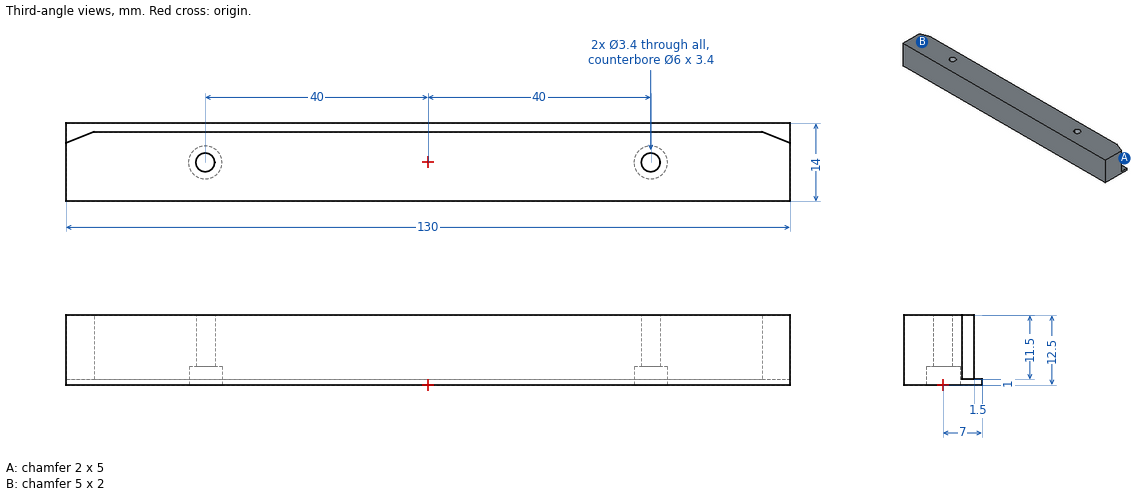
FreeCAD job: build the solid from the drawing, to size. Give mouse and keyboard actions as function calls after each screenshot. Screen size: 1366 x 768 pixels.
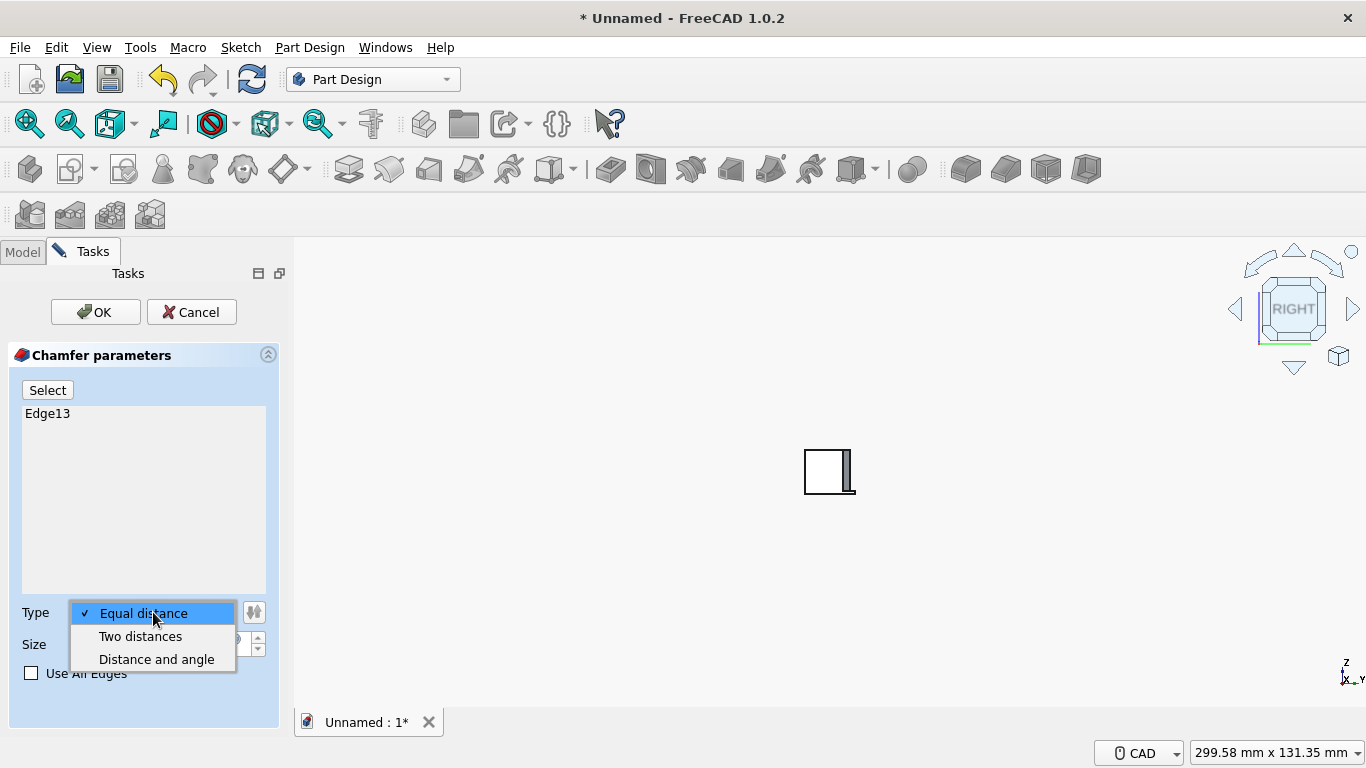
click(152, 636)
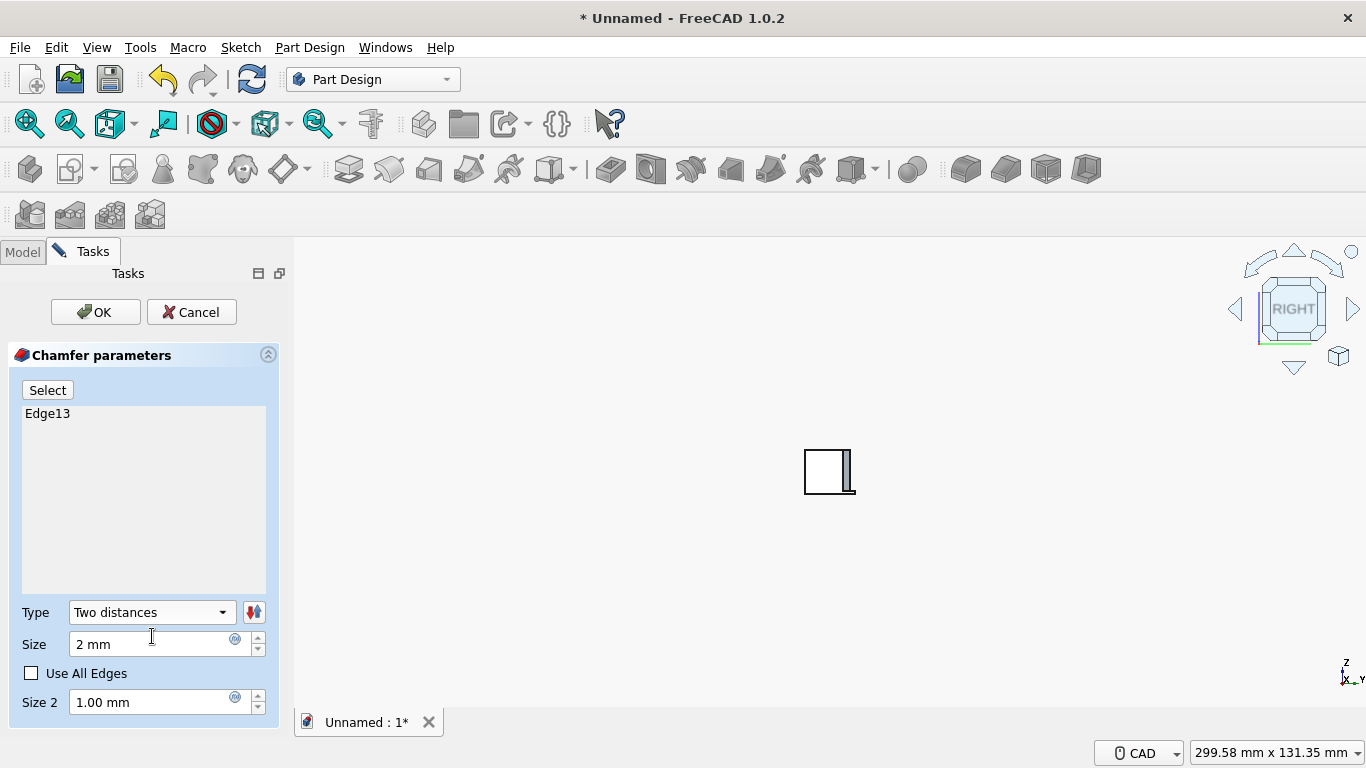
triple_click(160, 702)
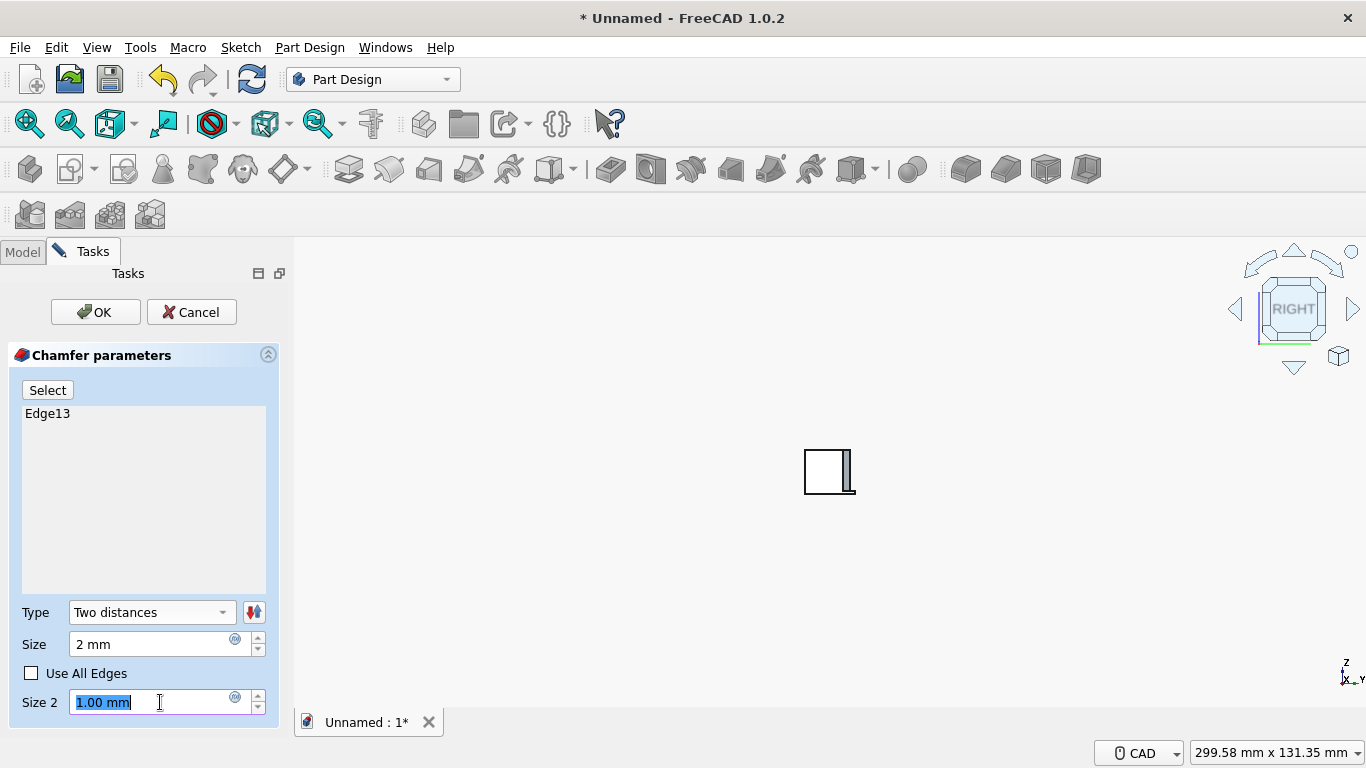
text(5)
key(Tab)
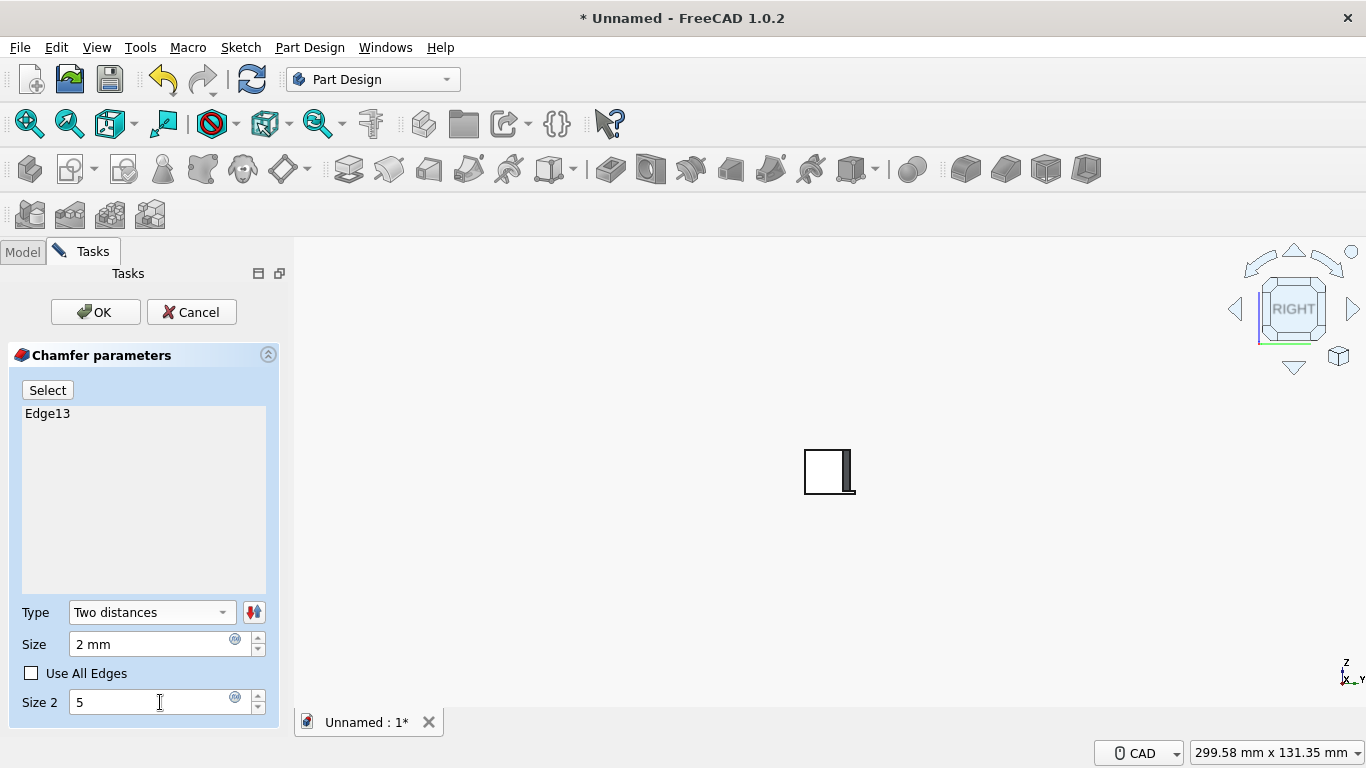
click(96, 312)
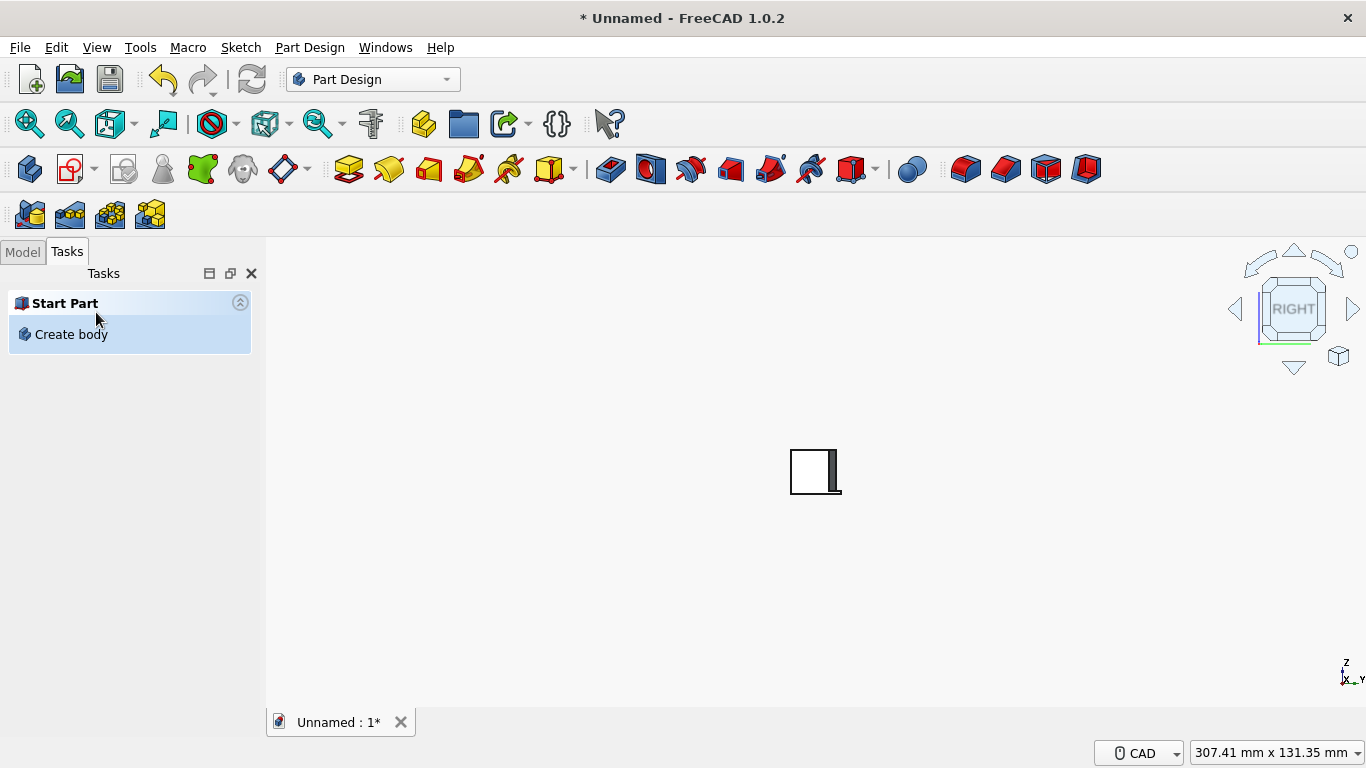
click(30, 124)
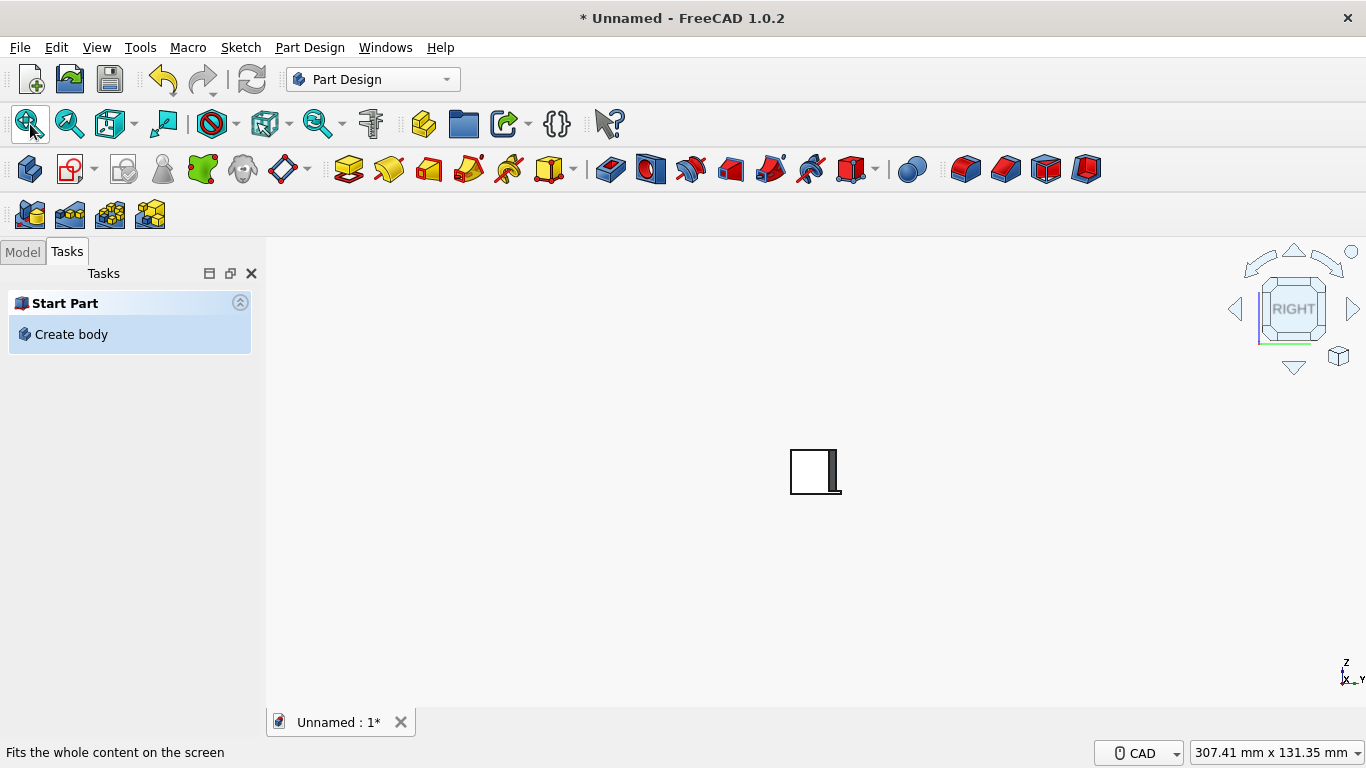
key(0)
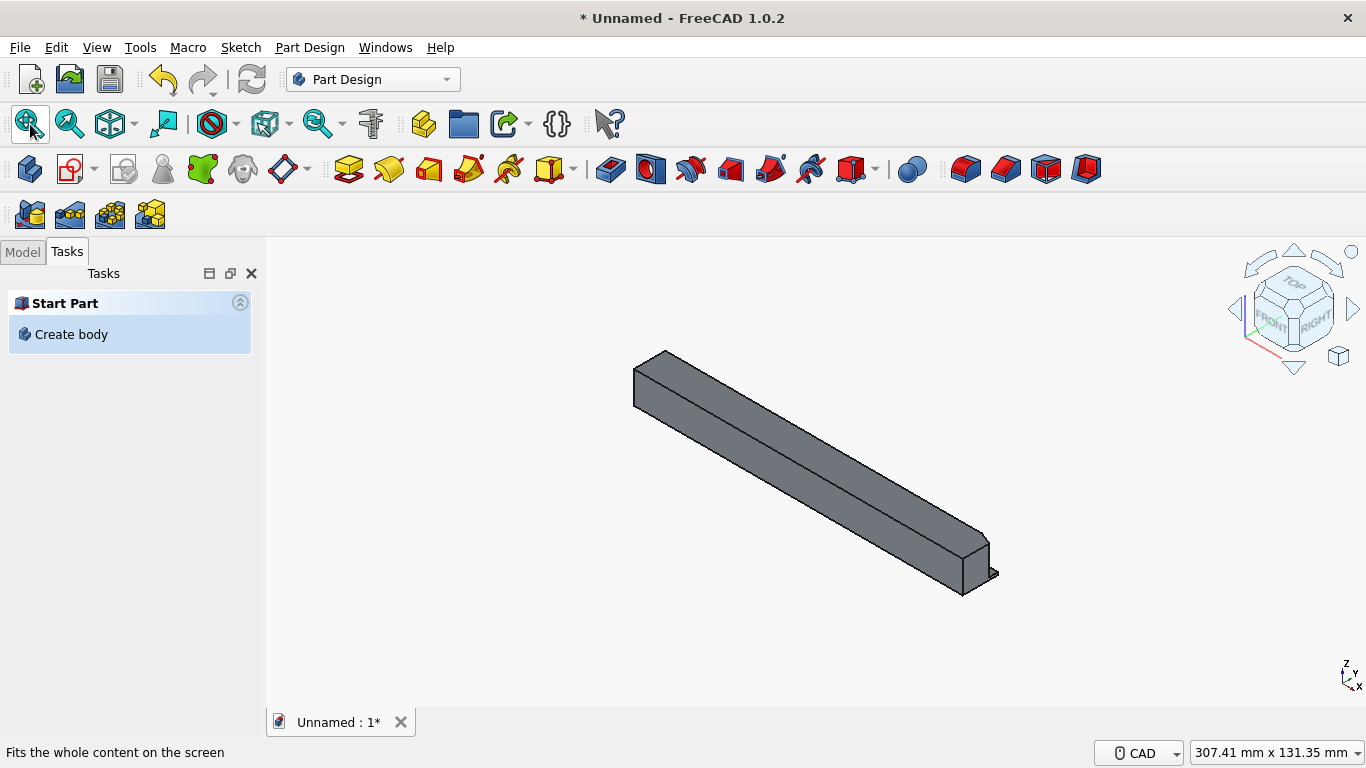
key(2)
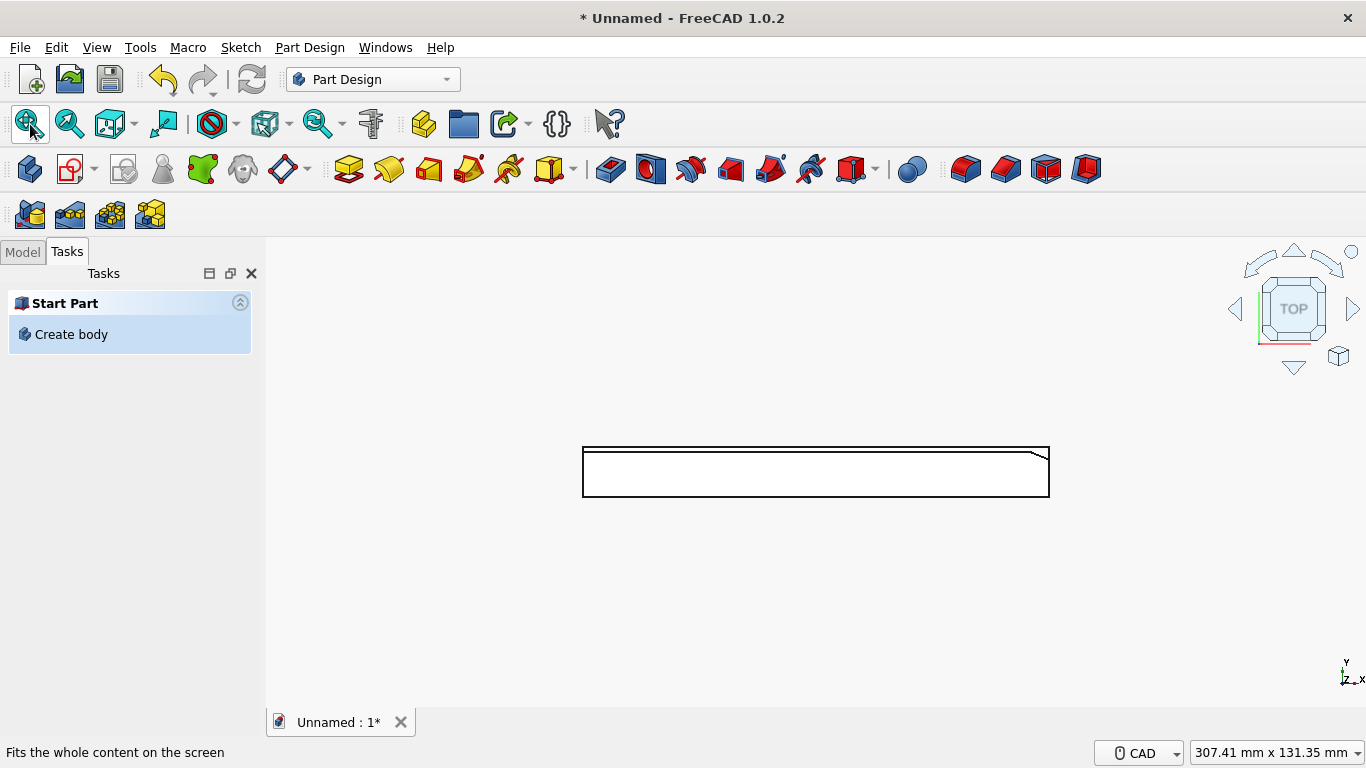
click(30, 124)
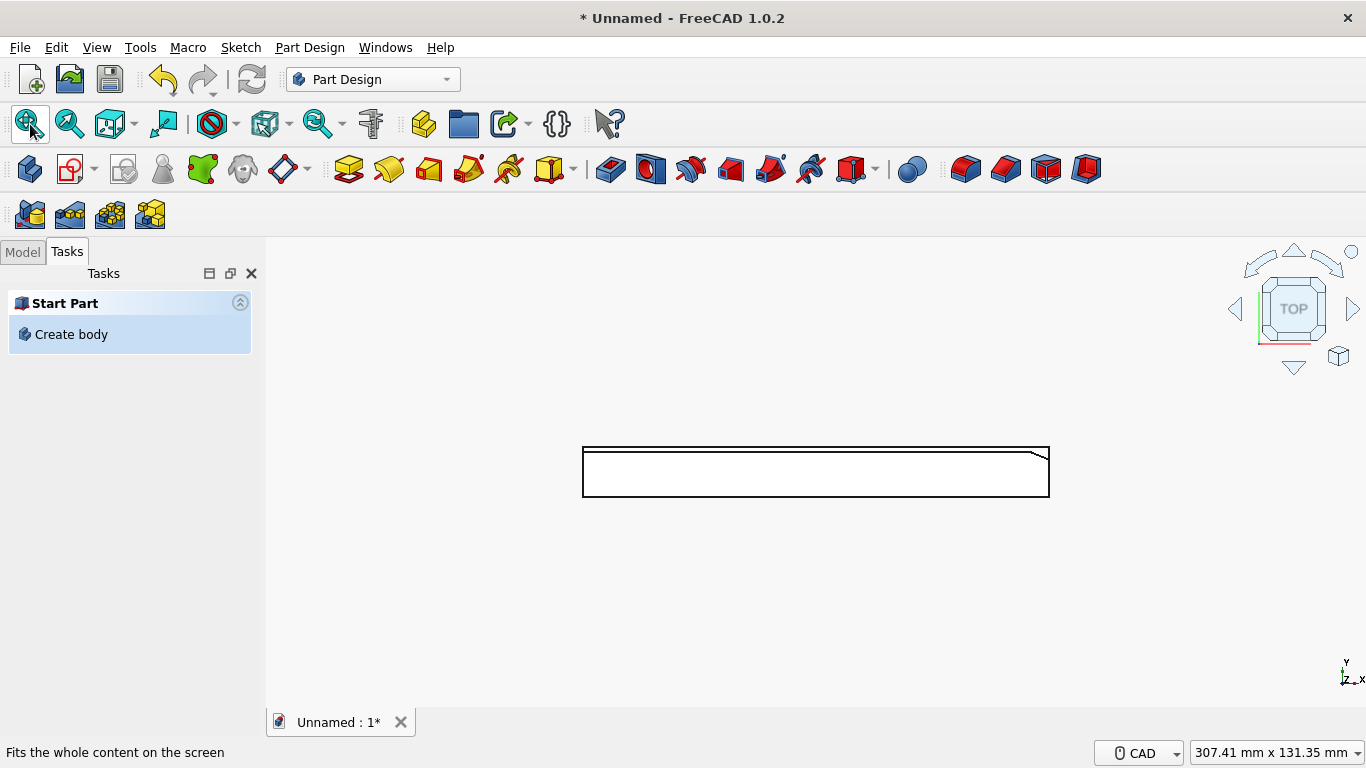
key(1)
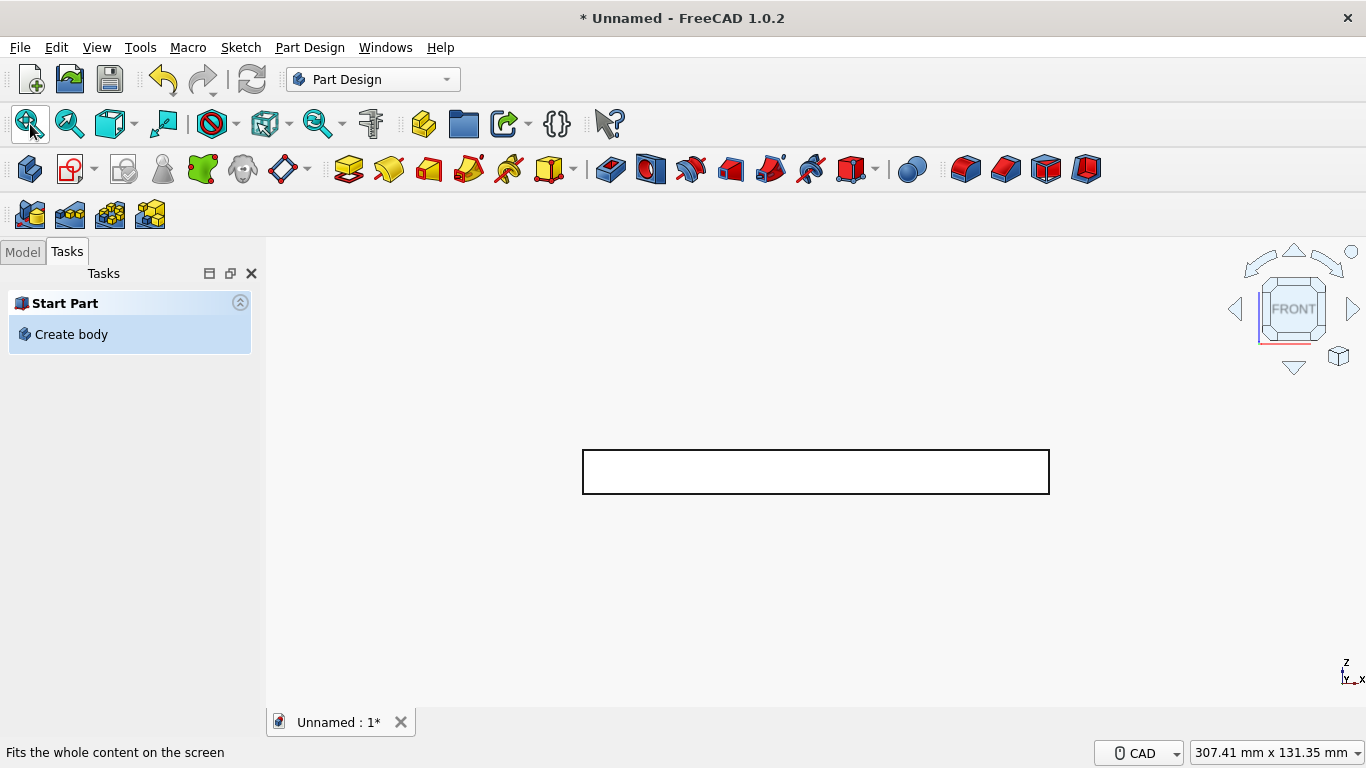
click(30, 124)